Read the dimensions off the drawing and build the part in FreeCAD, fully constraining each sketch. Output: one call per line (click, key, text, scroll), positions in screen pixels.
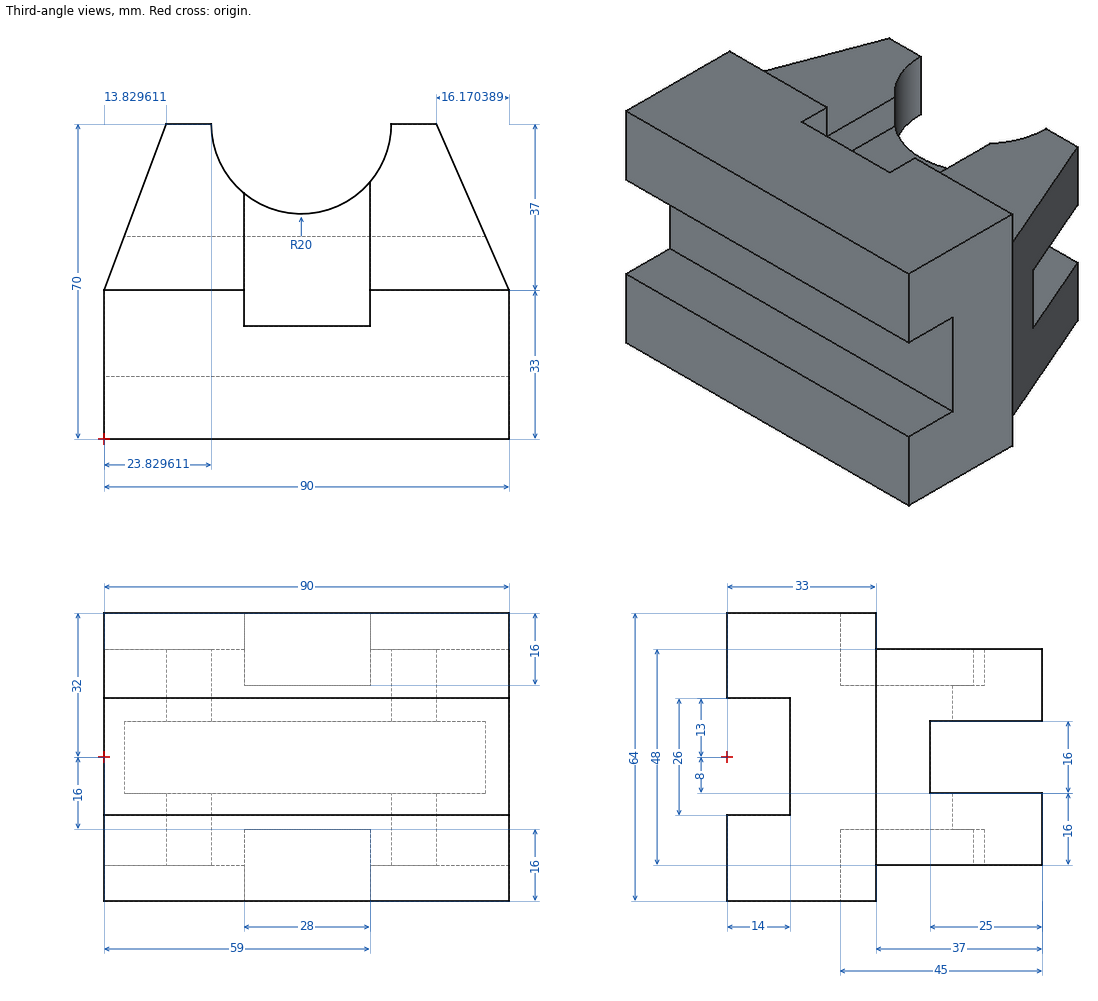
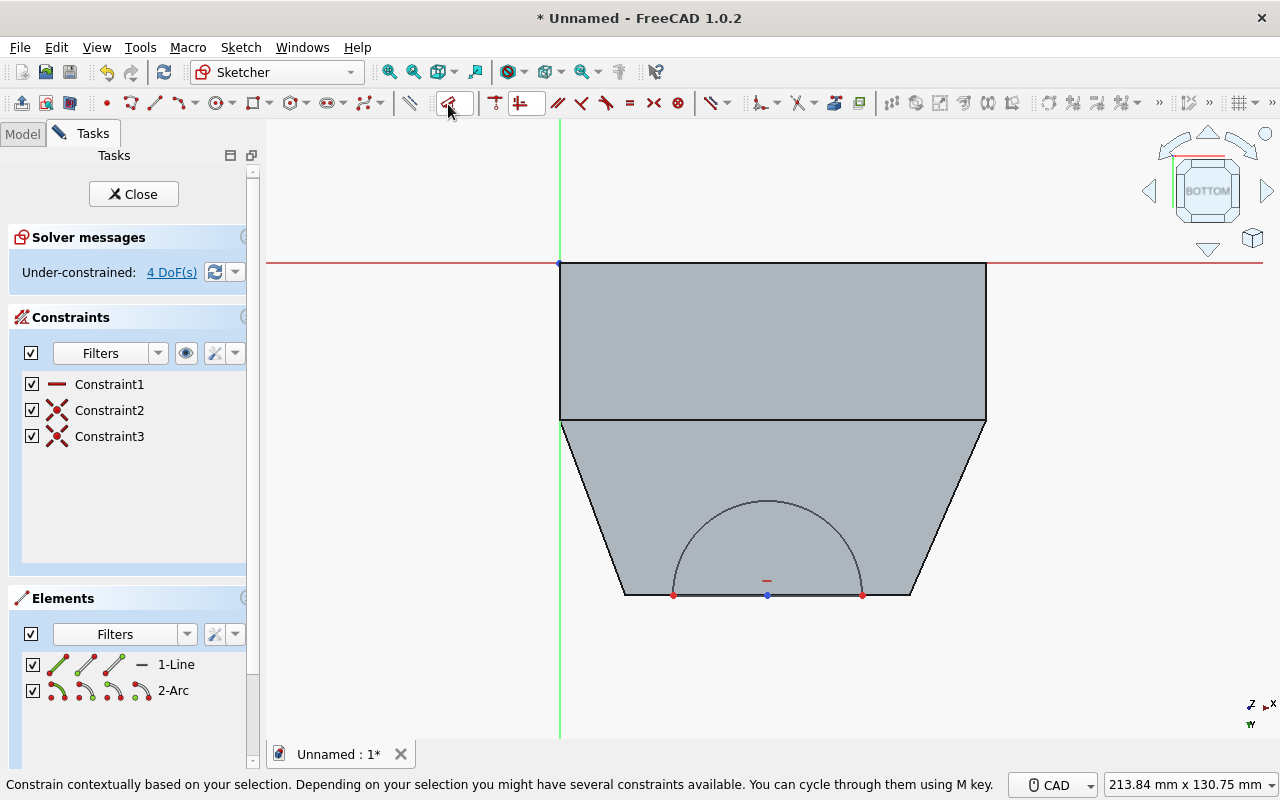
click(823, 519)
click(842, 493)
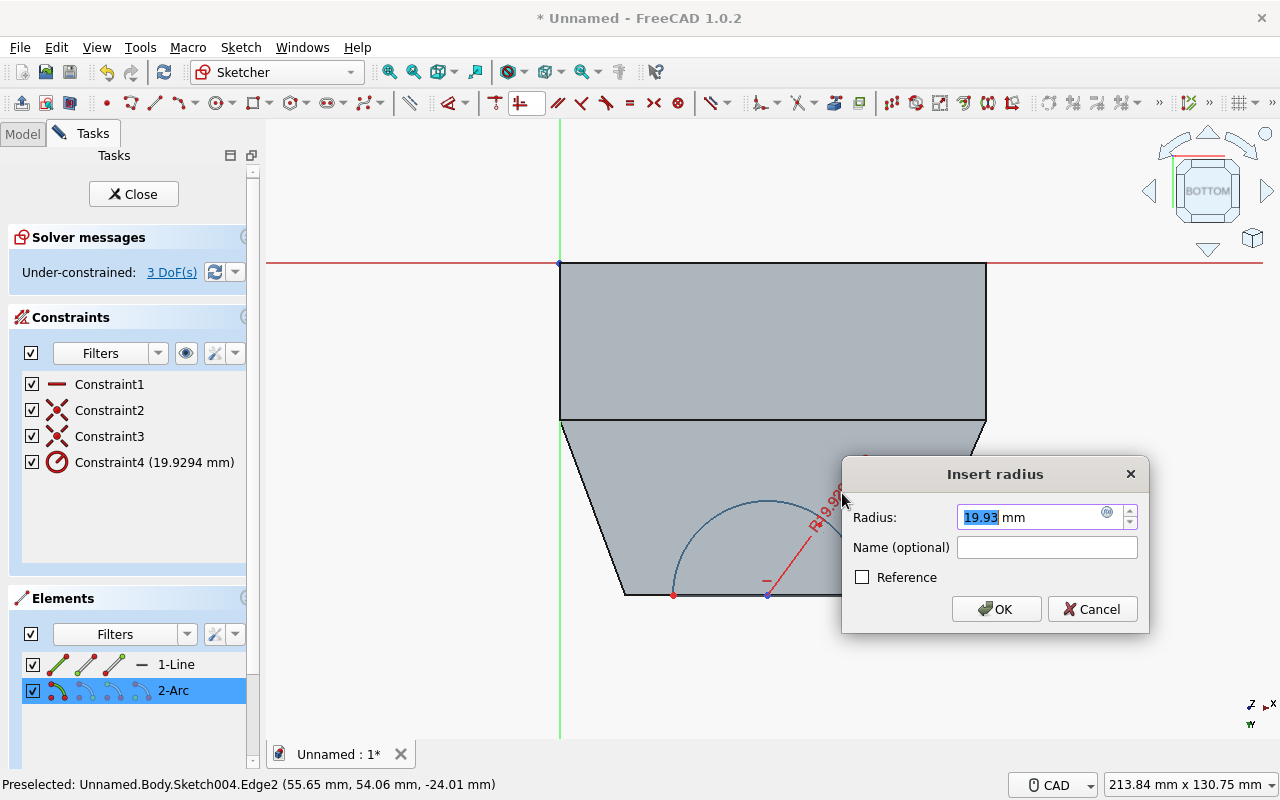
text(20)
key(Return)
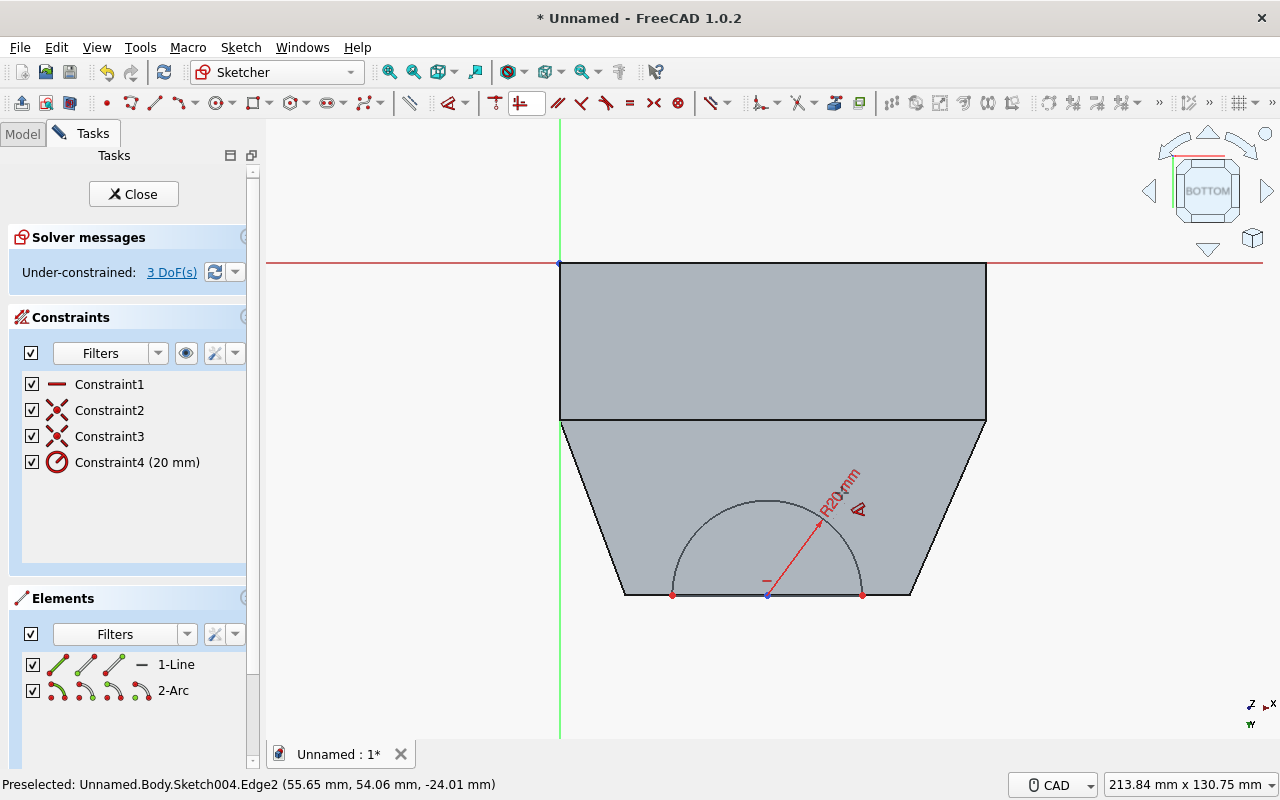
click(672, 596)
click(526, 430)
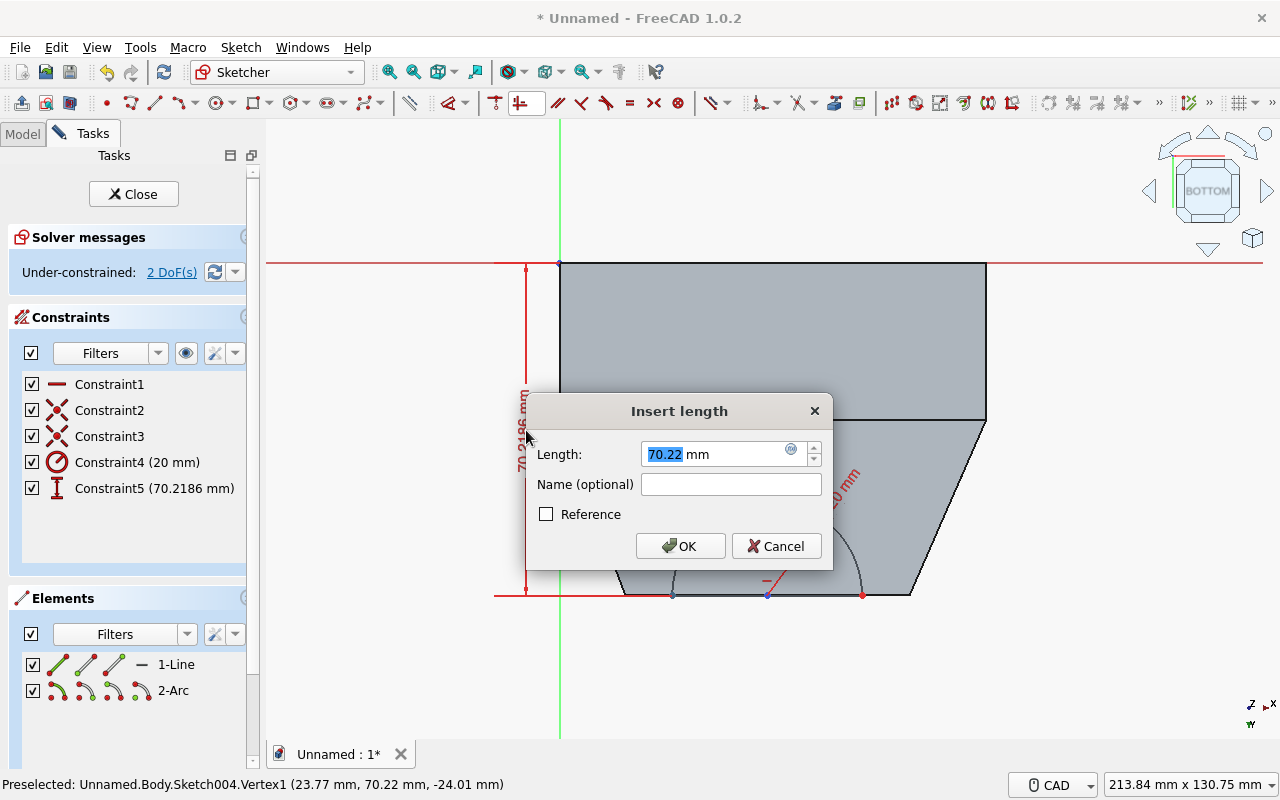
text(70)
key(Return)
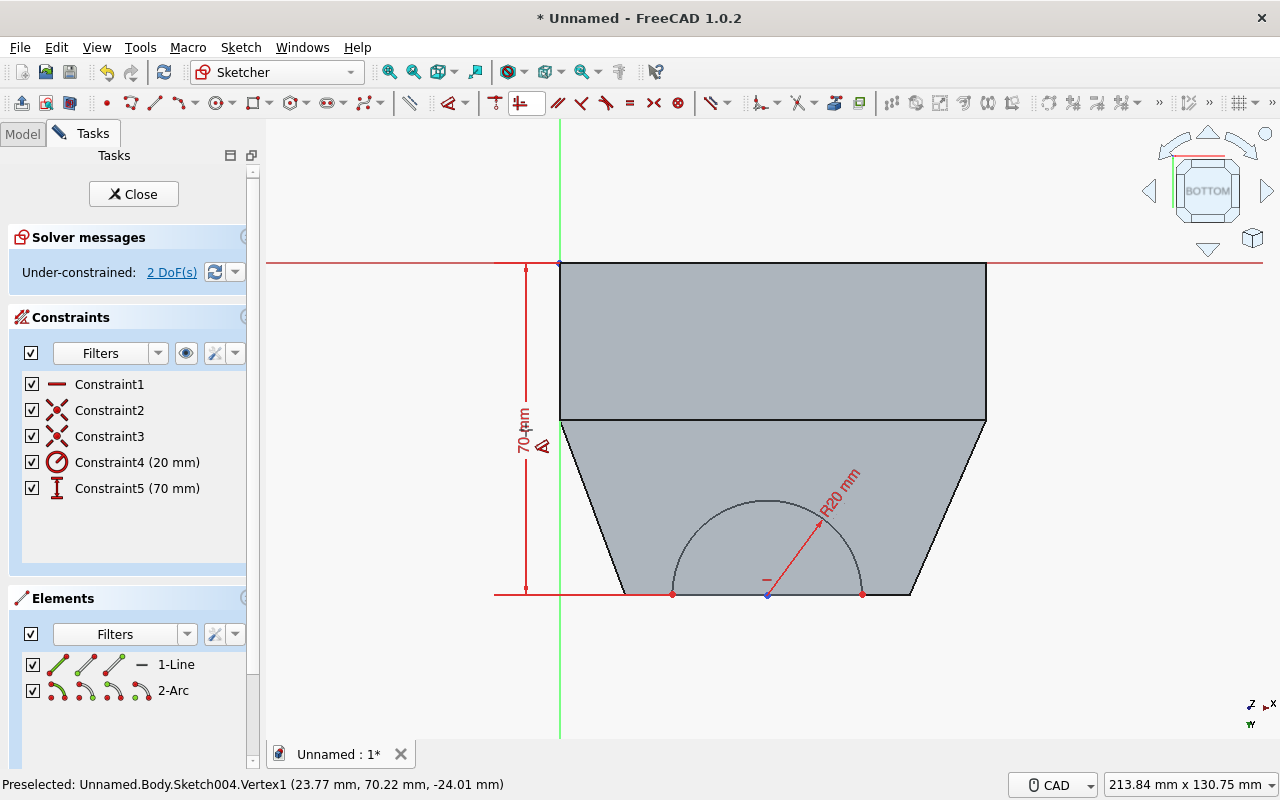
click(767, 596)
click(526, 353)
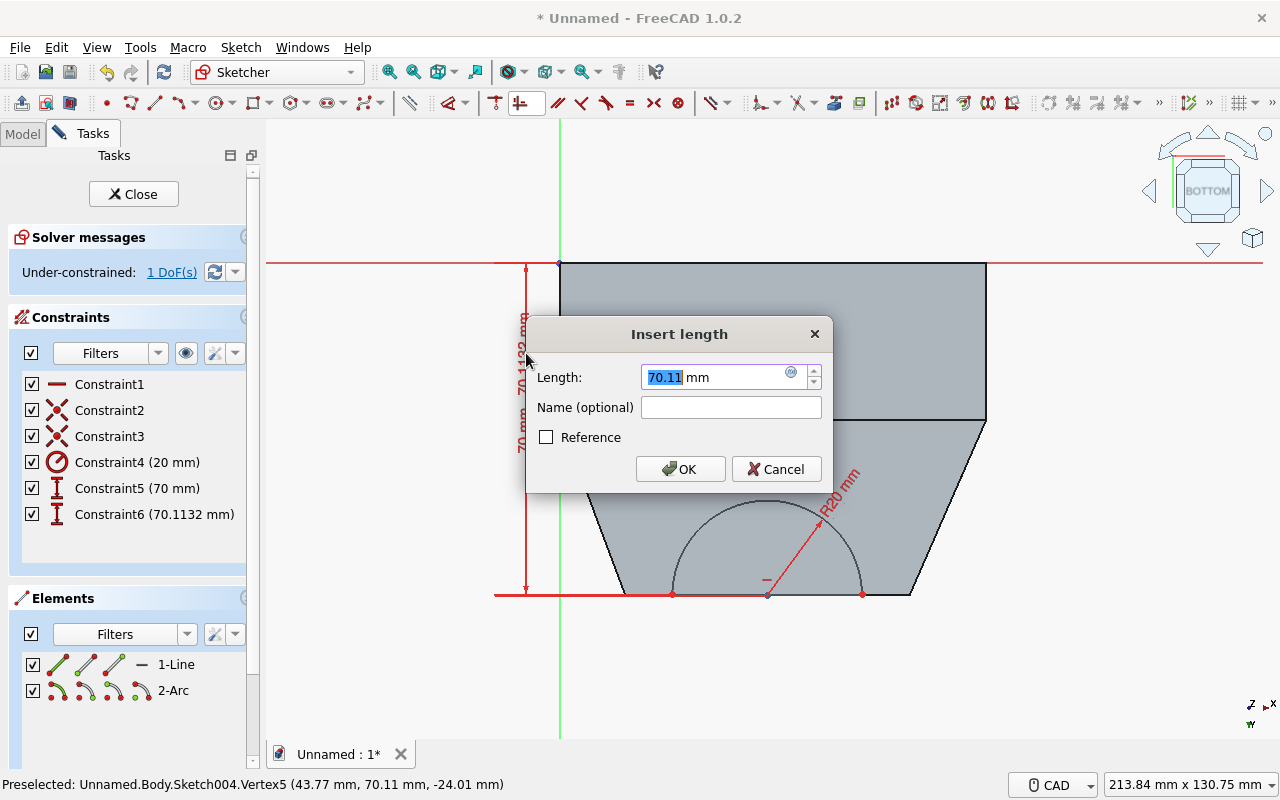
text(70)
key(Return)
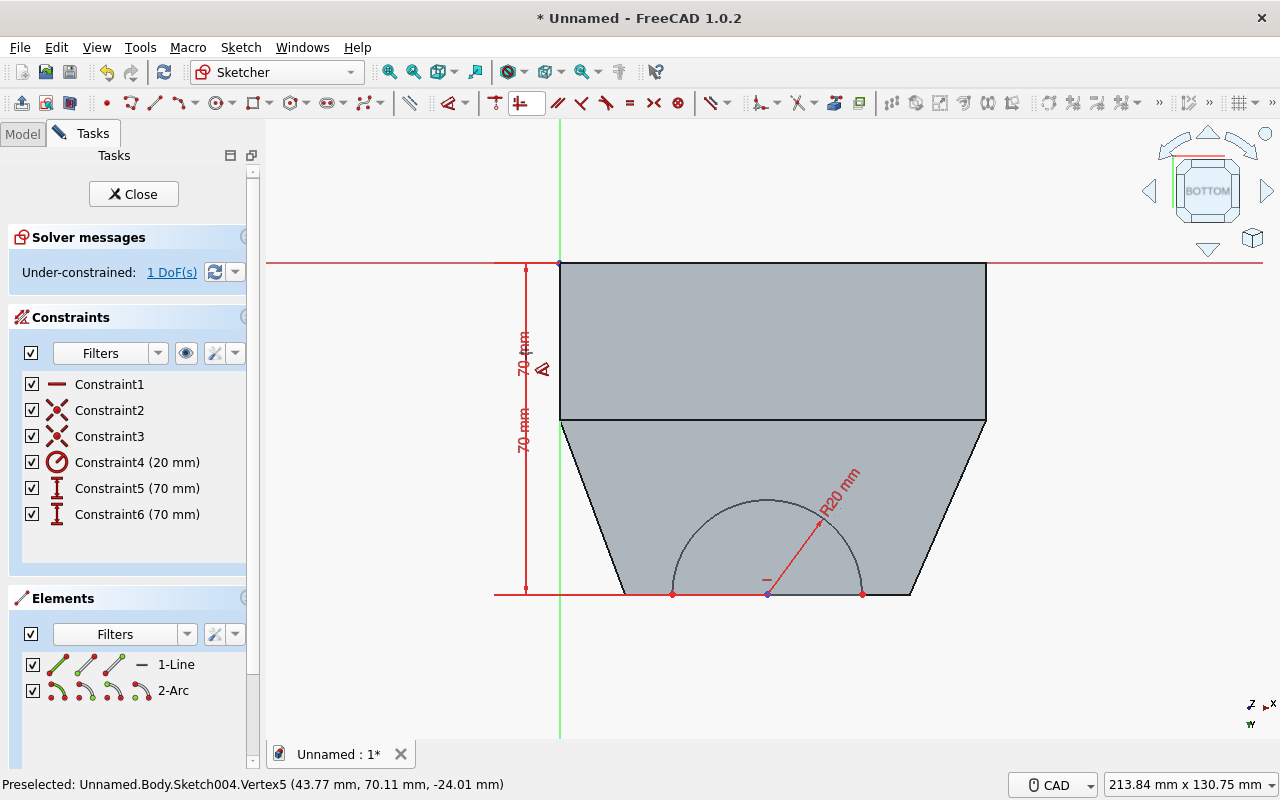
click(672, 595)
click(616, 629)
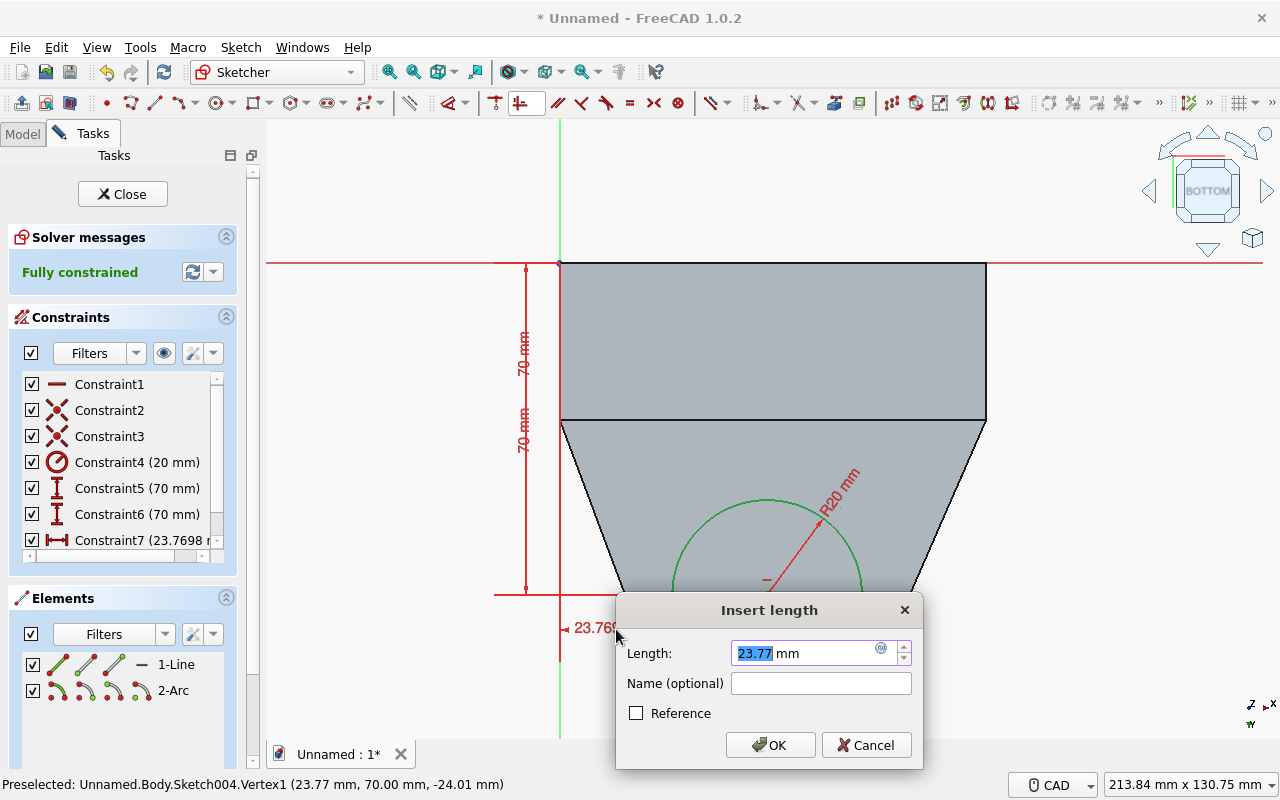
text(23.829611)
key(Return)
key(Escape)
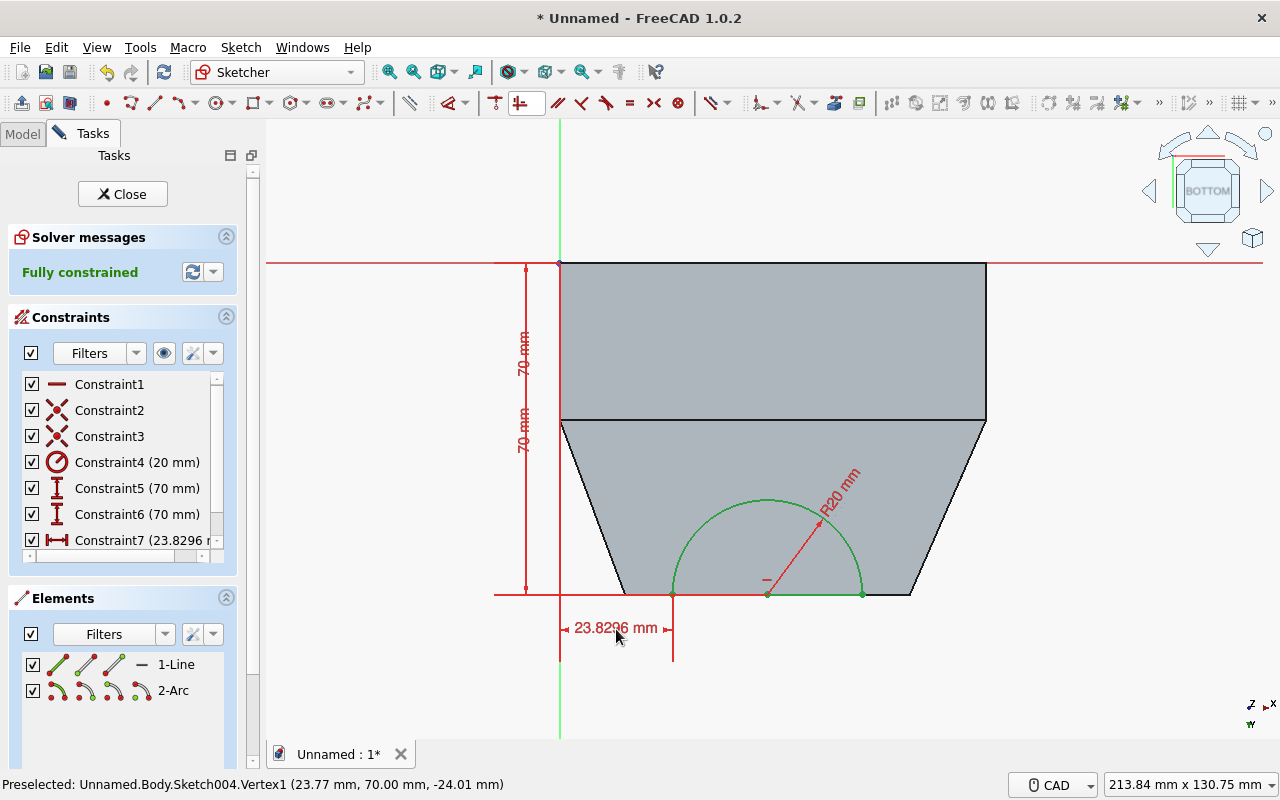
click(123, 194)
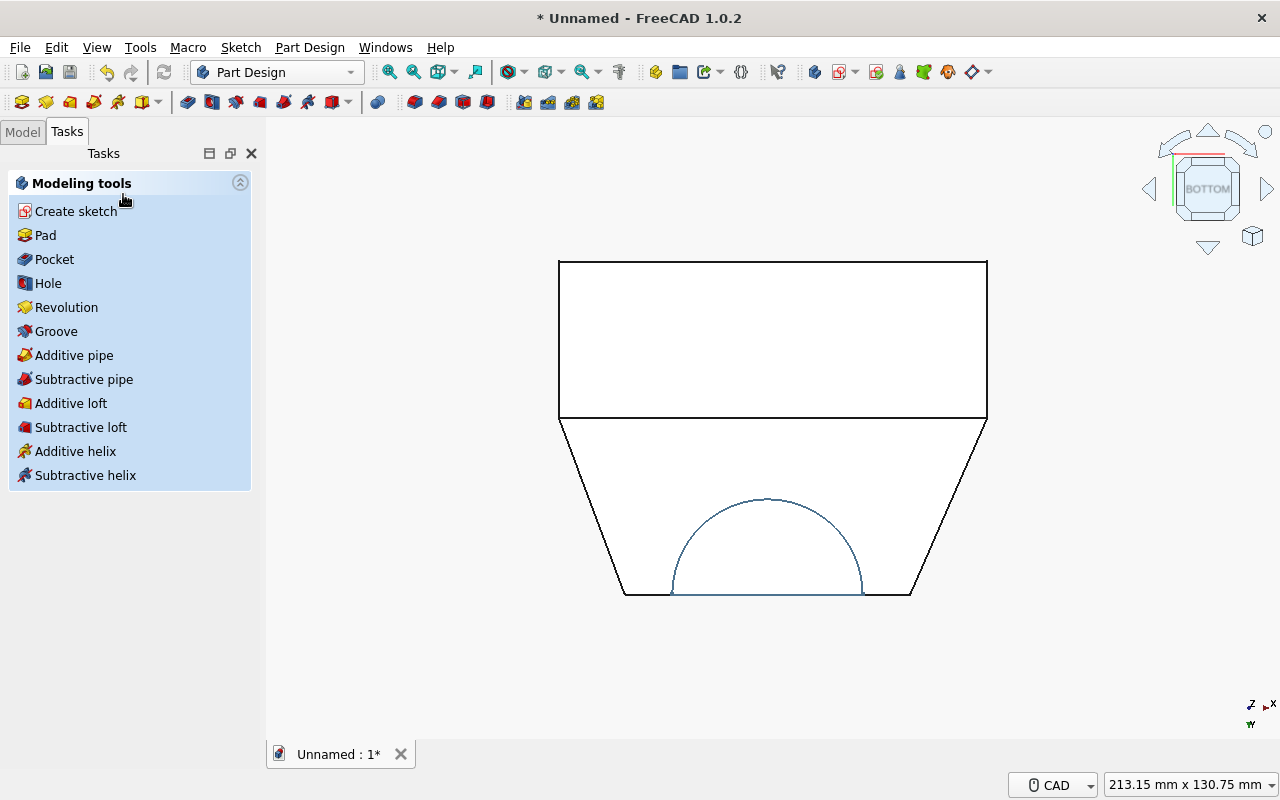
click(188, 102)